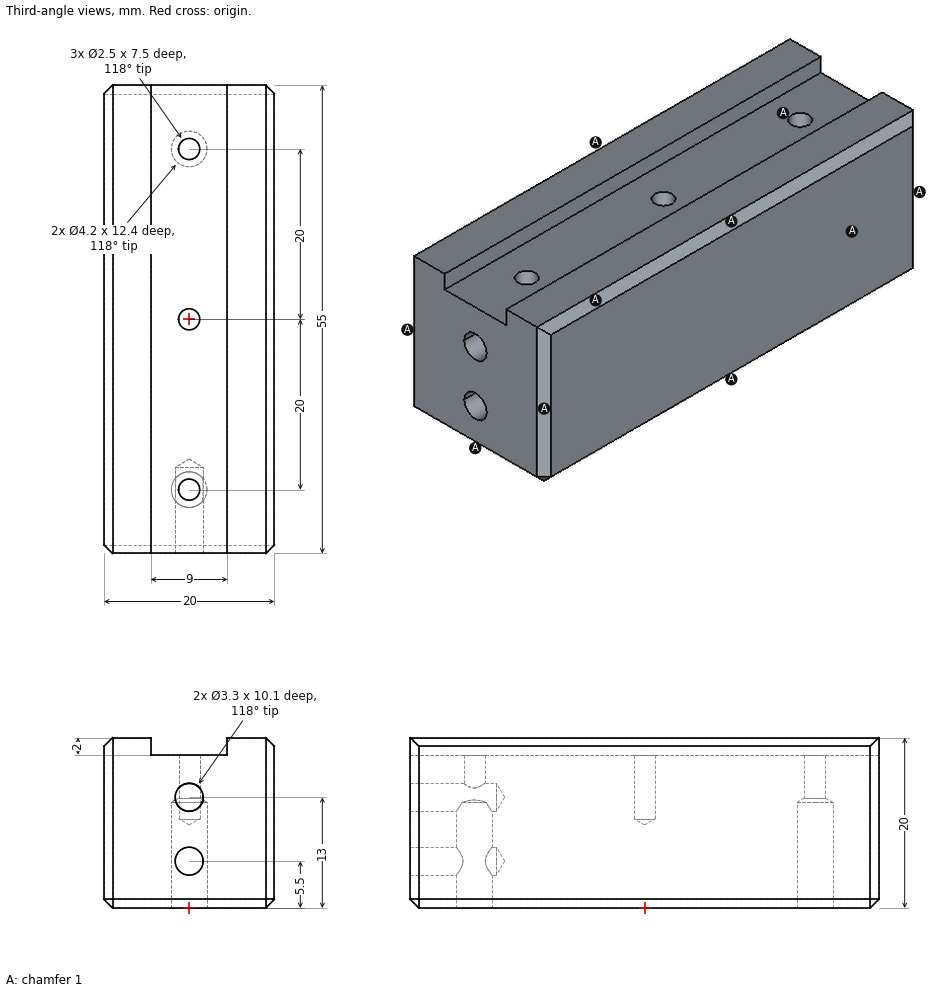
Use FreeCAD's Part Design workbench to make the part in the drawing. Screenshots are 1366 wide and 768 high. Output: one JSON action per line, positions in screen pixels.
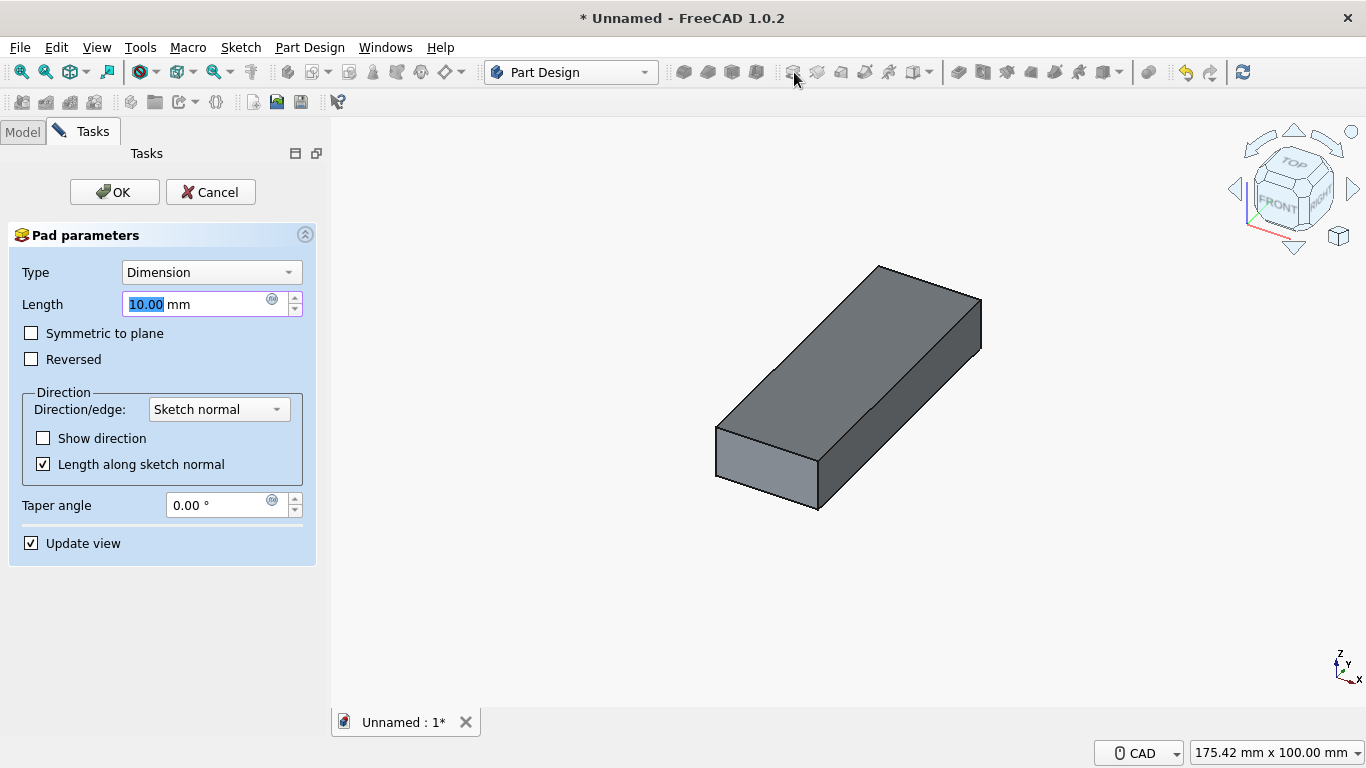
{"action": "type", "text": "20"}
{"action": "key", "text": "Tab"}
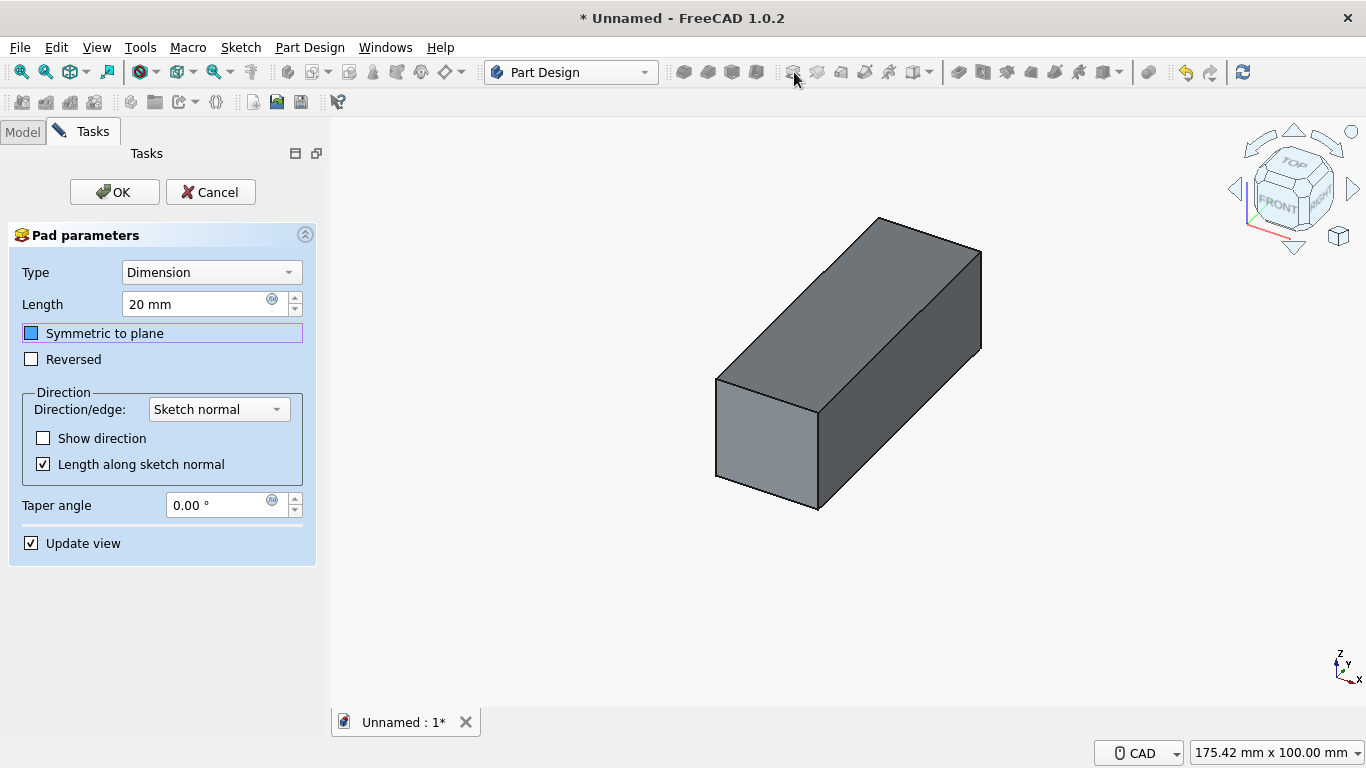
{"action": "left_click", "coordinate": [115, 192]}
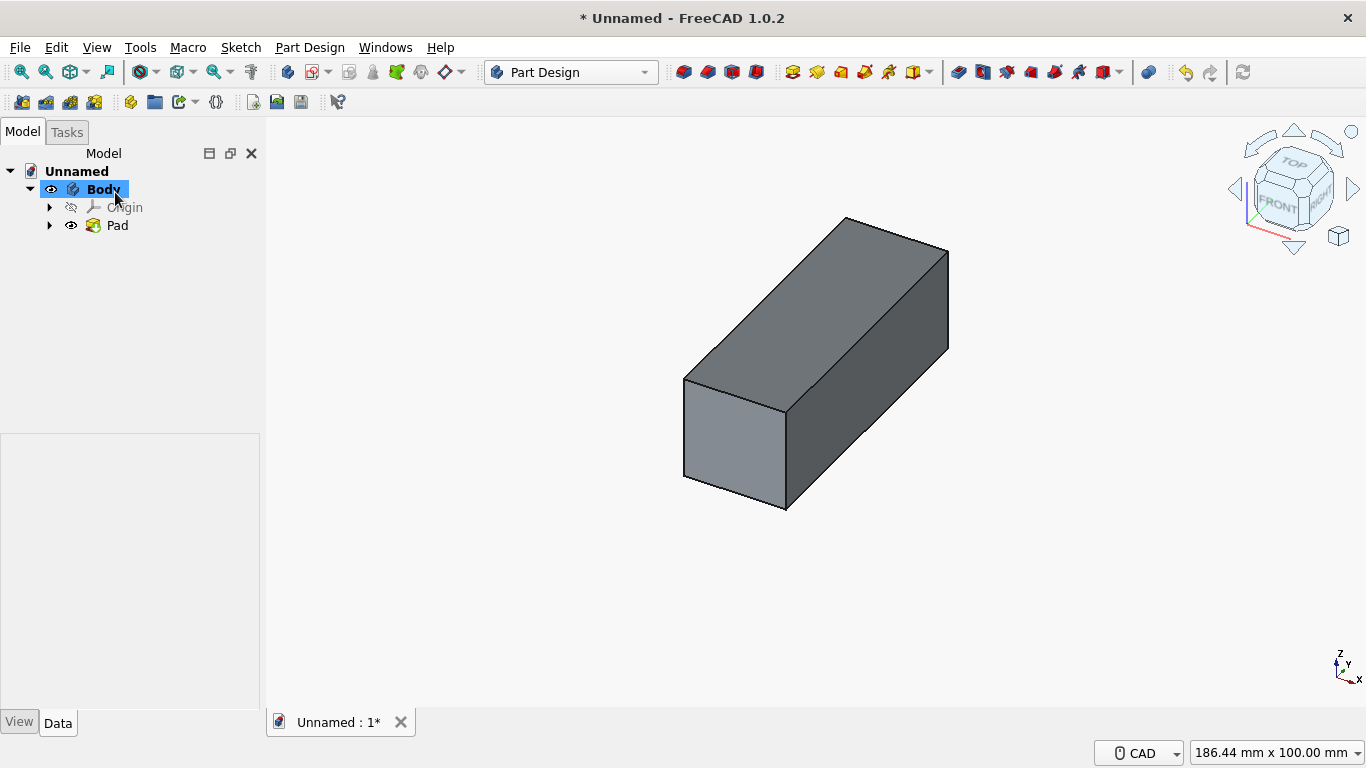
{"action": "left_click", "coordinate": [862, 268]}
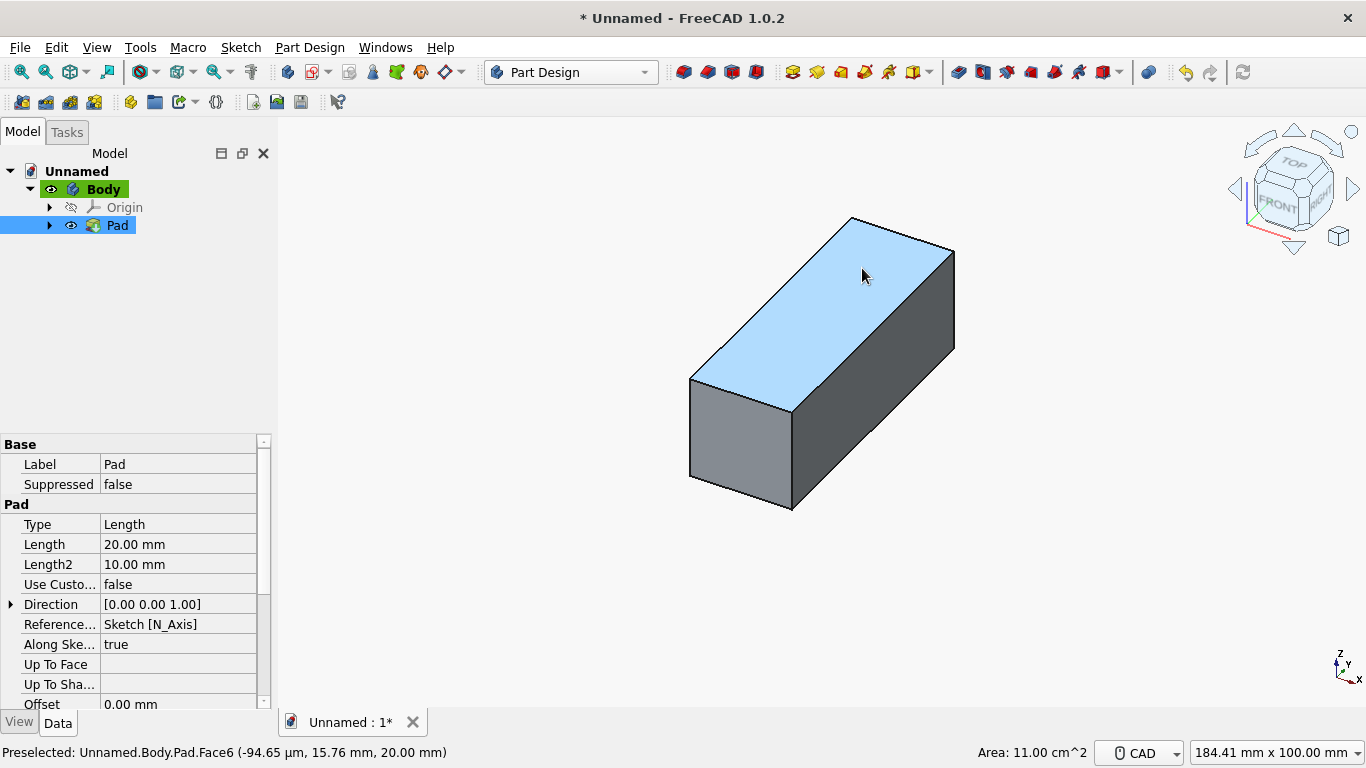
{"action": "left_click", "coordinate": [312, 72]}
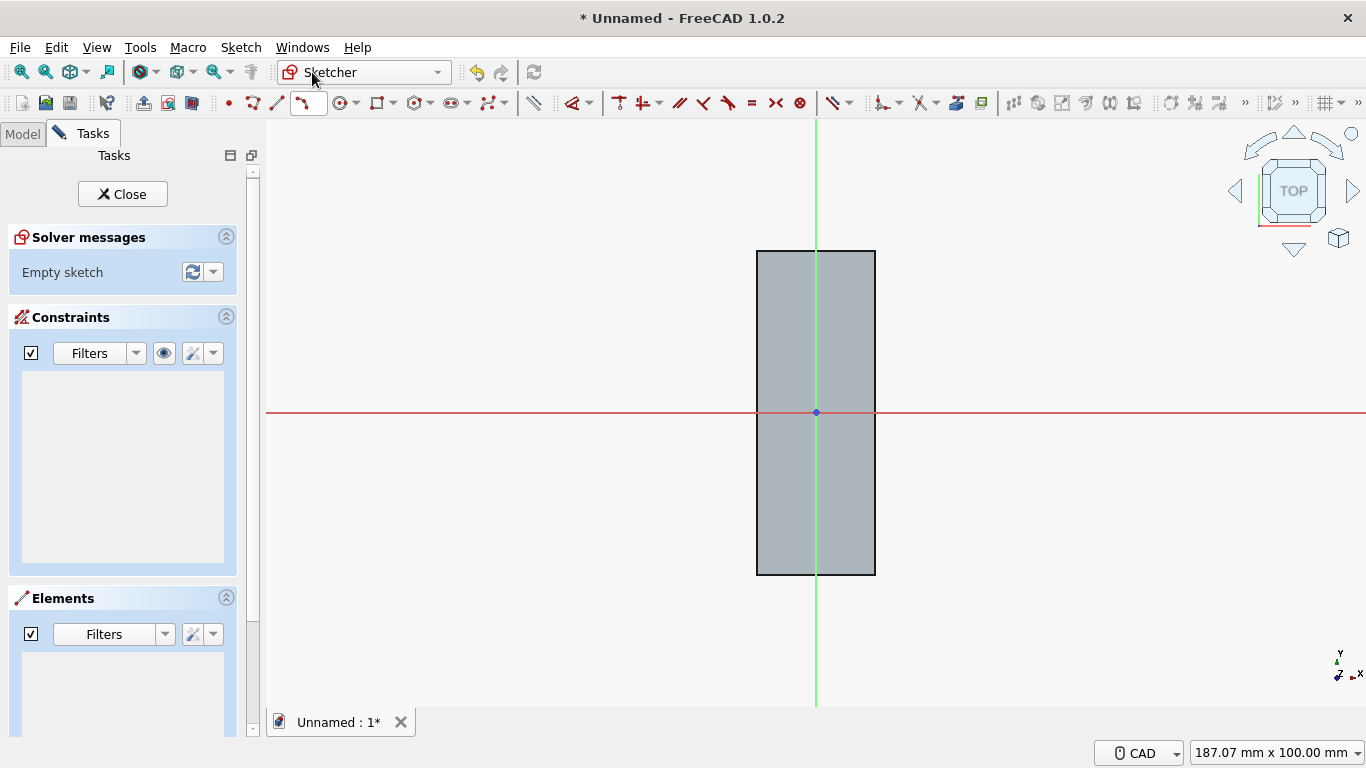
{"action": "left_click", "coordinate": [396, 104]}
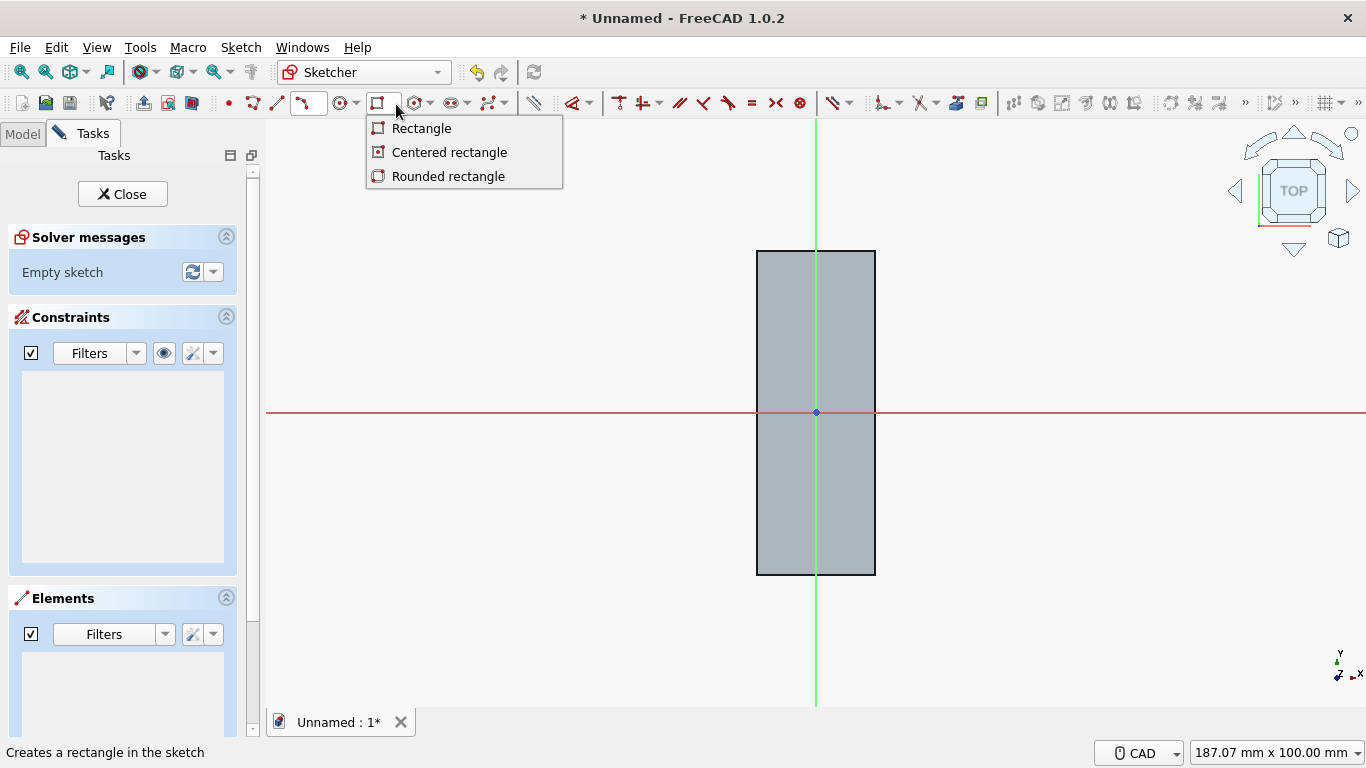
{"action": "left_click", "coordinate": [464, 152]}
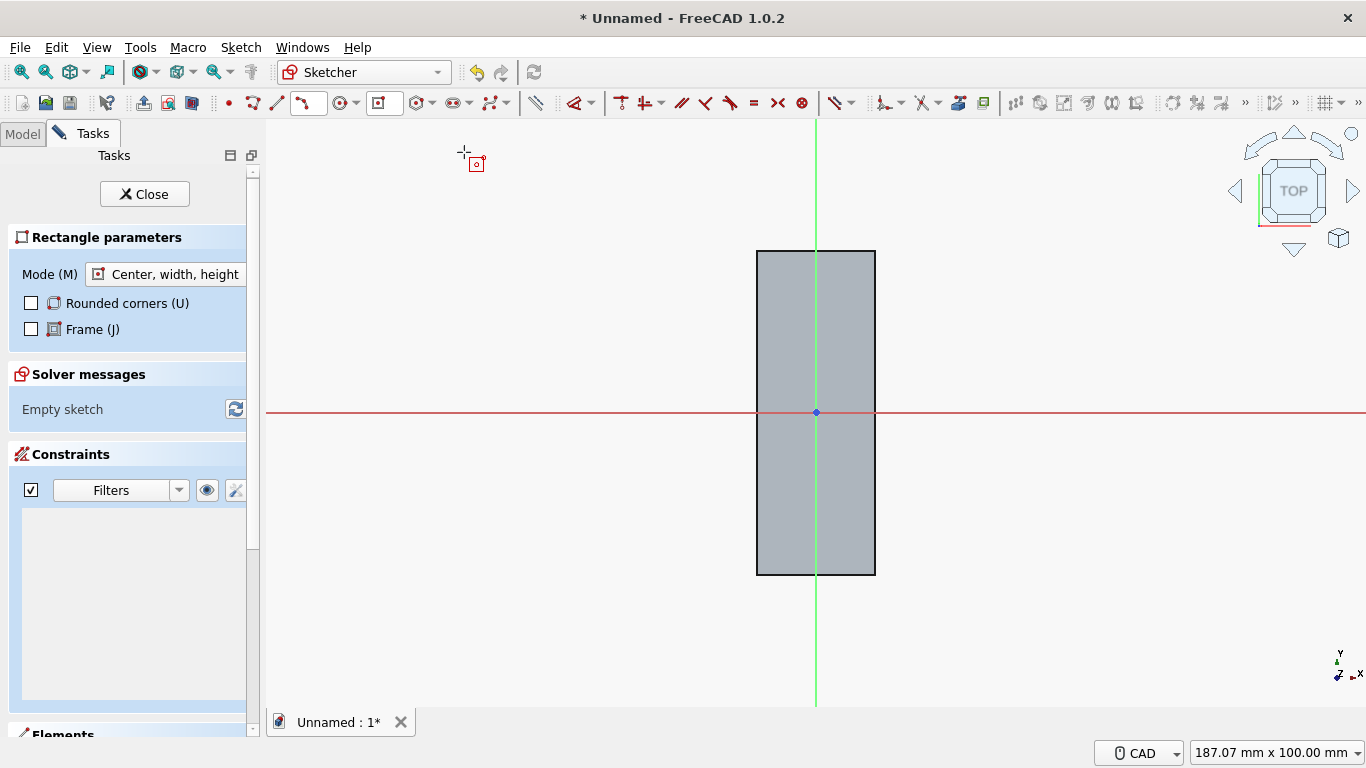
{"action": "left_click", "coordinate": [816, 413]}
{"action": "mouse_move", "coordinate": [842, 251]}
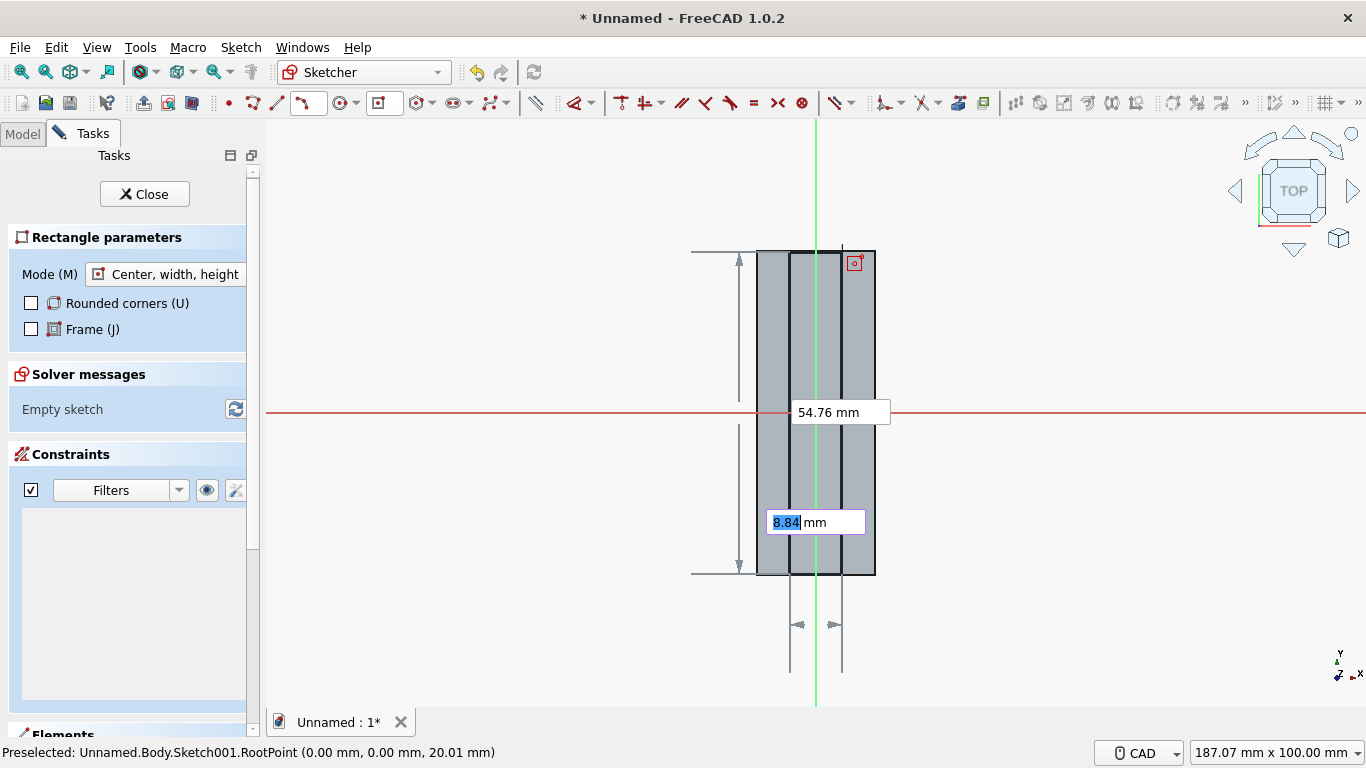
{"action": "type", "text": "9"}
{"action": "key", "text": "Tab"}
{"action": "type", "text": "55"}
{"action": "key", "text": "Return"}
{"action": "key", "text": "Escape"}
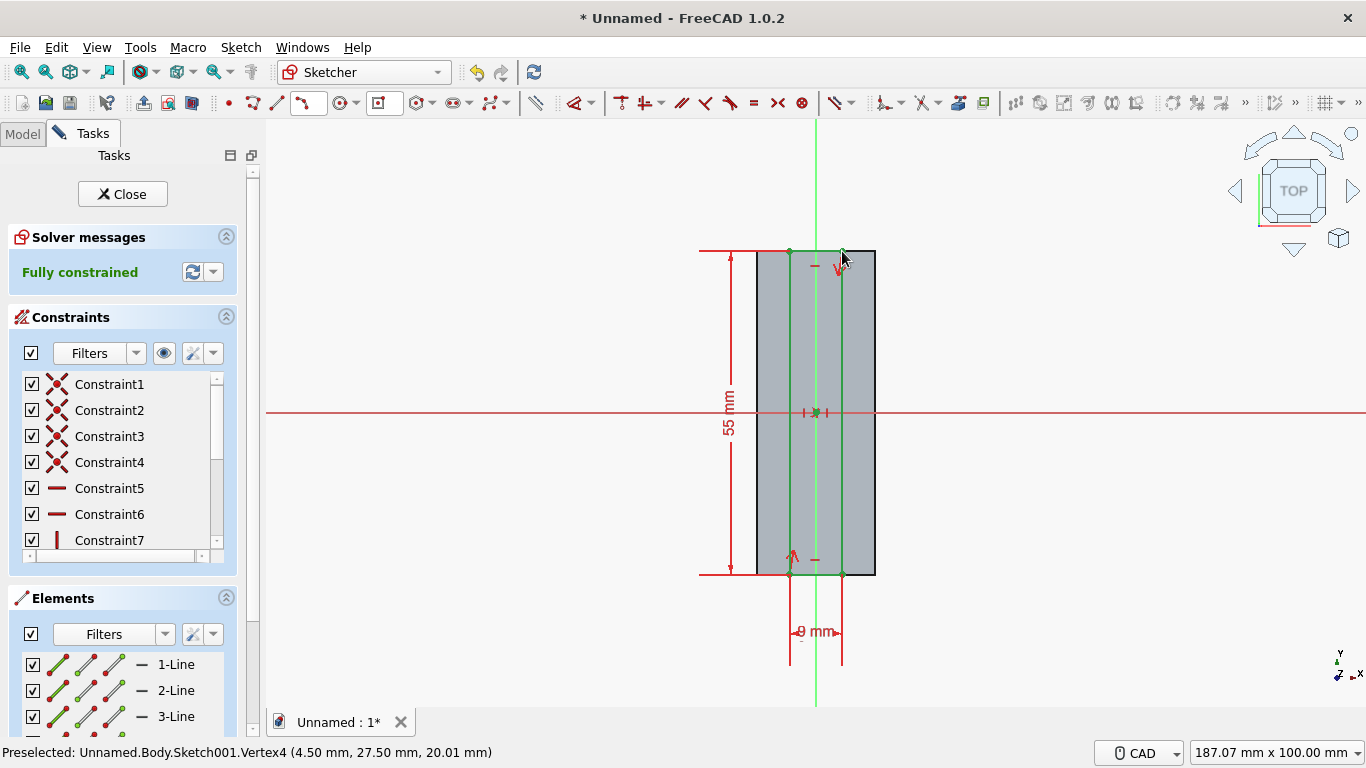
{"action": "left_click", "coordinate": [123, 194]}